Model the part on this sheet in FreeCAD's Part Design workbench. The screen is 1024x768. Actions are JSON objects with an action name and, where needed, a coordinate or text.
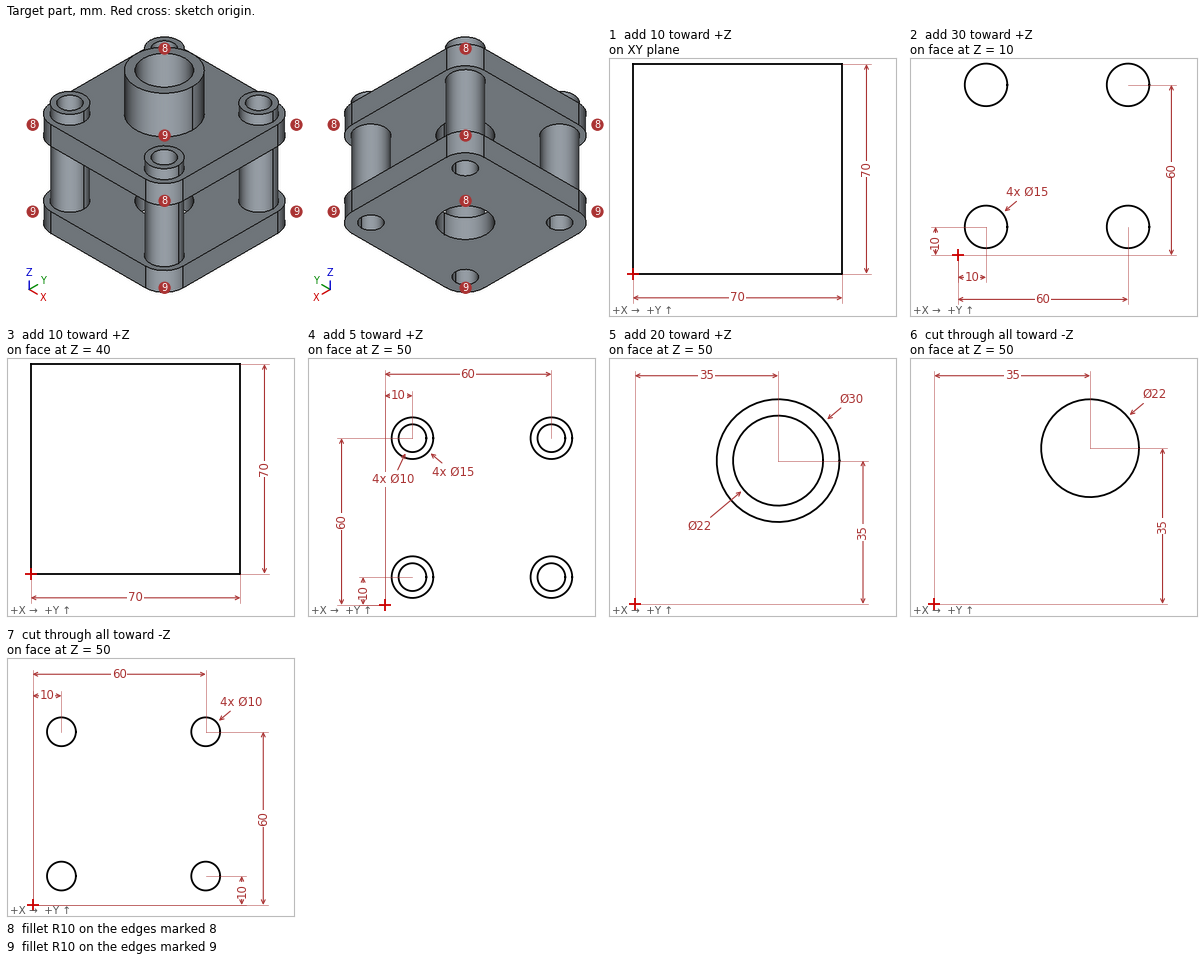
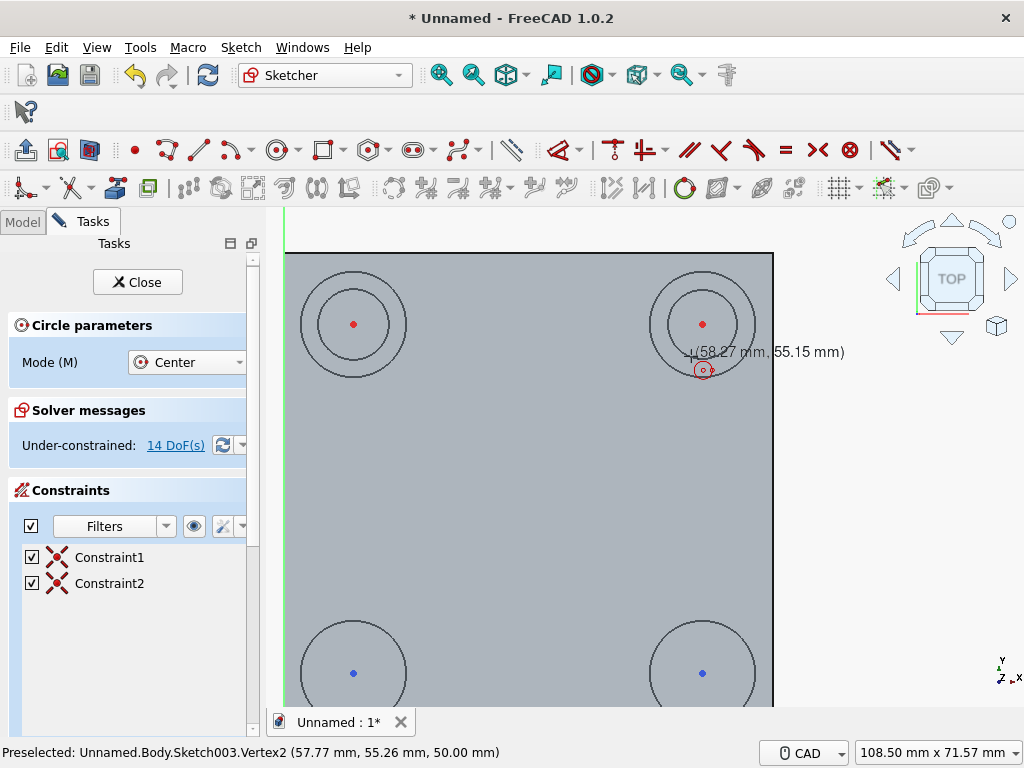
{"action": "left_click", "coordinate": [353, 674]}
{"action": "left_click", "coordinate": [378, 648]}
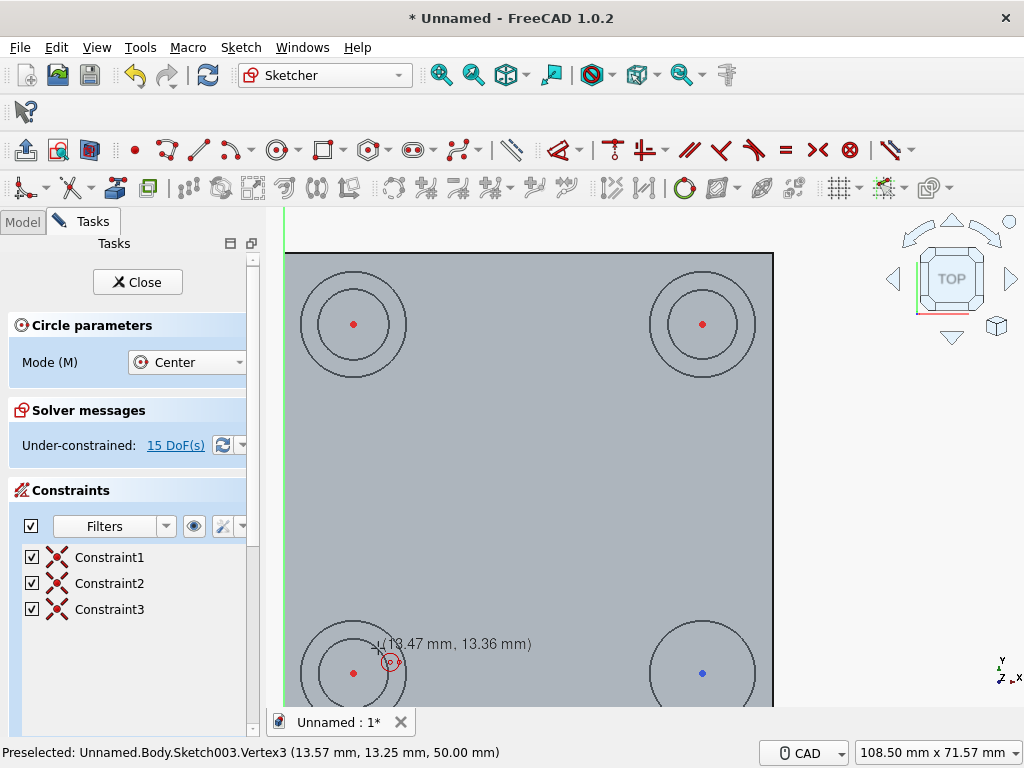
{"action": "left_click", "coordinate": [702, 674]}
{"action": "left_click", "coordinate": [728, 648]}
{"action": "key", "text": "Escape"}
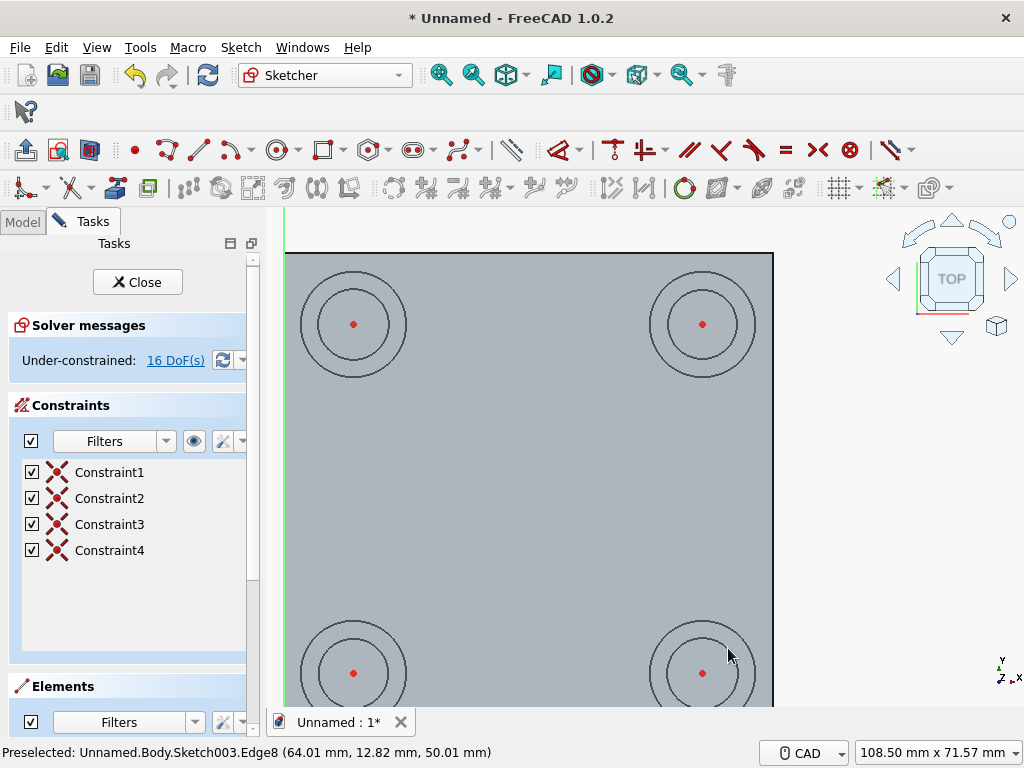
{"action": "left_click", "coordinate": [391, 287]}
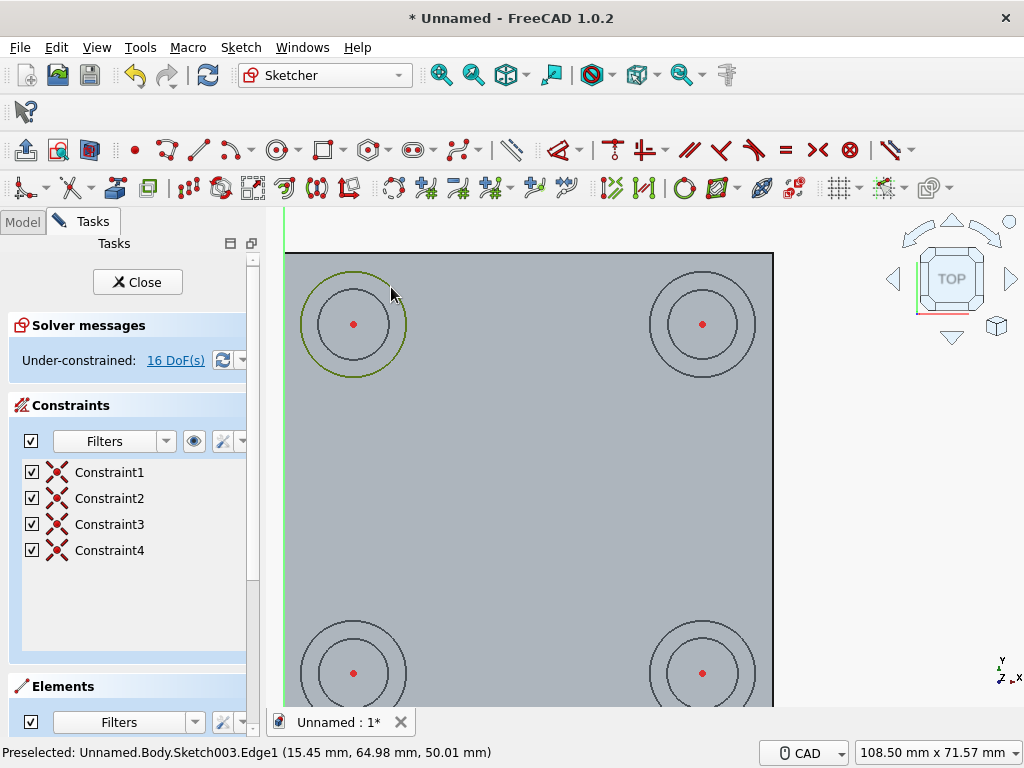
{"action": "left_click", "coordinate": [740, 287]}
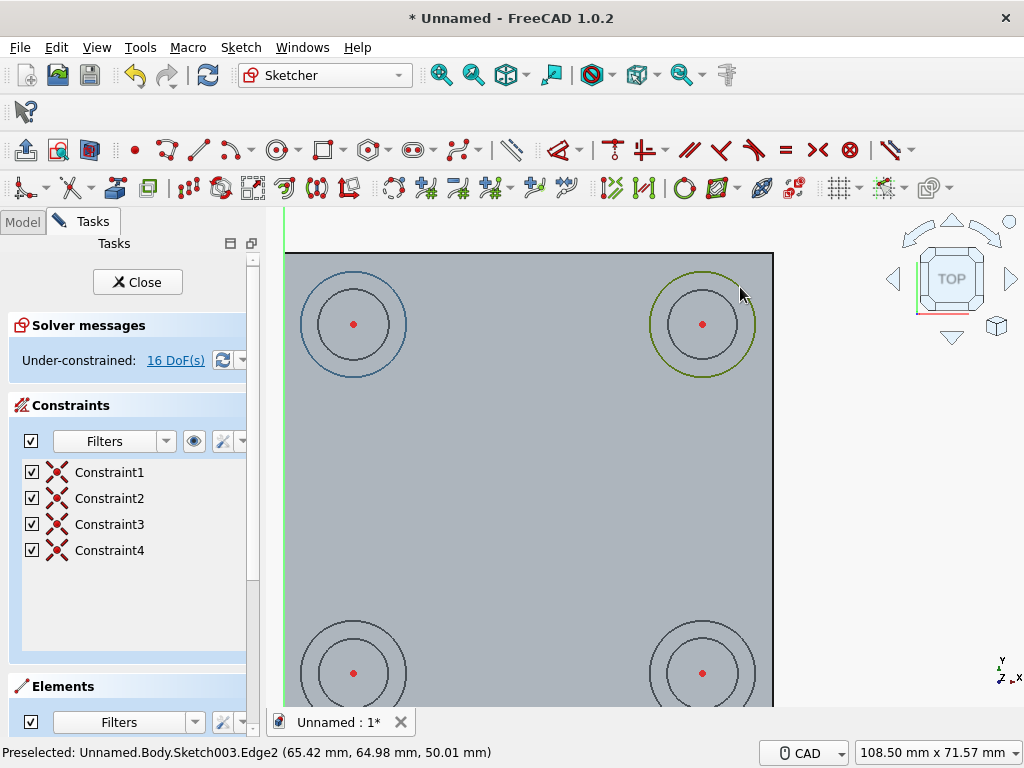
{"action": "left_click", "coordinate": [391, 636]}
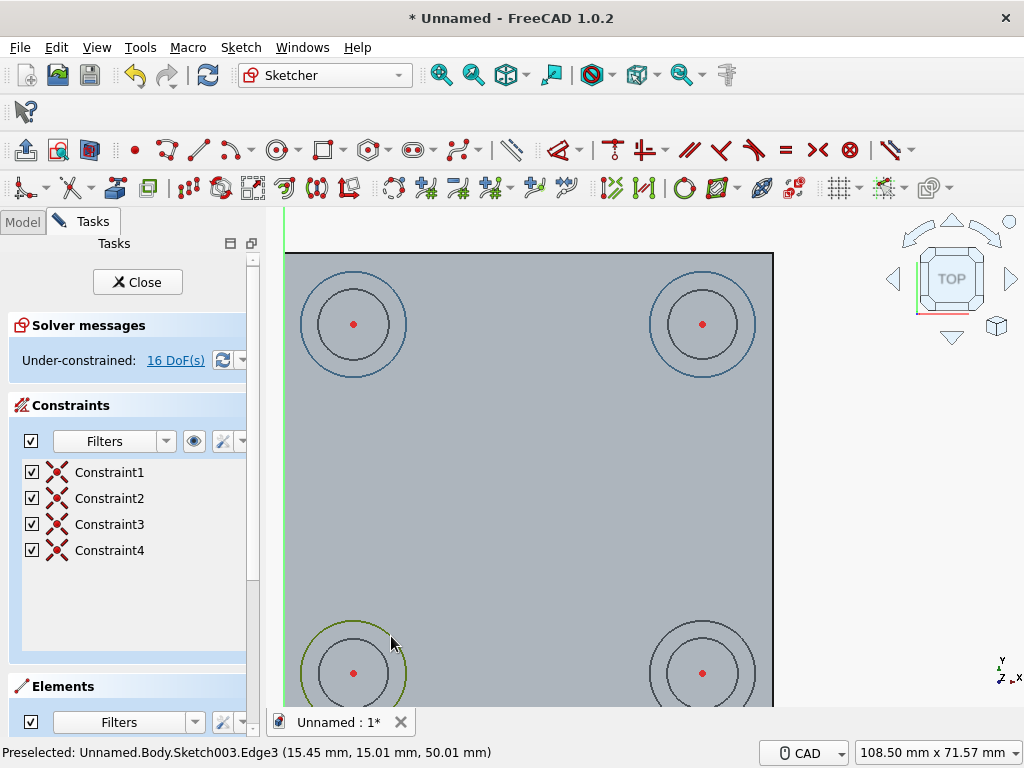
{"action": "left_click", "coordinate": [740, 636]}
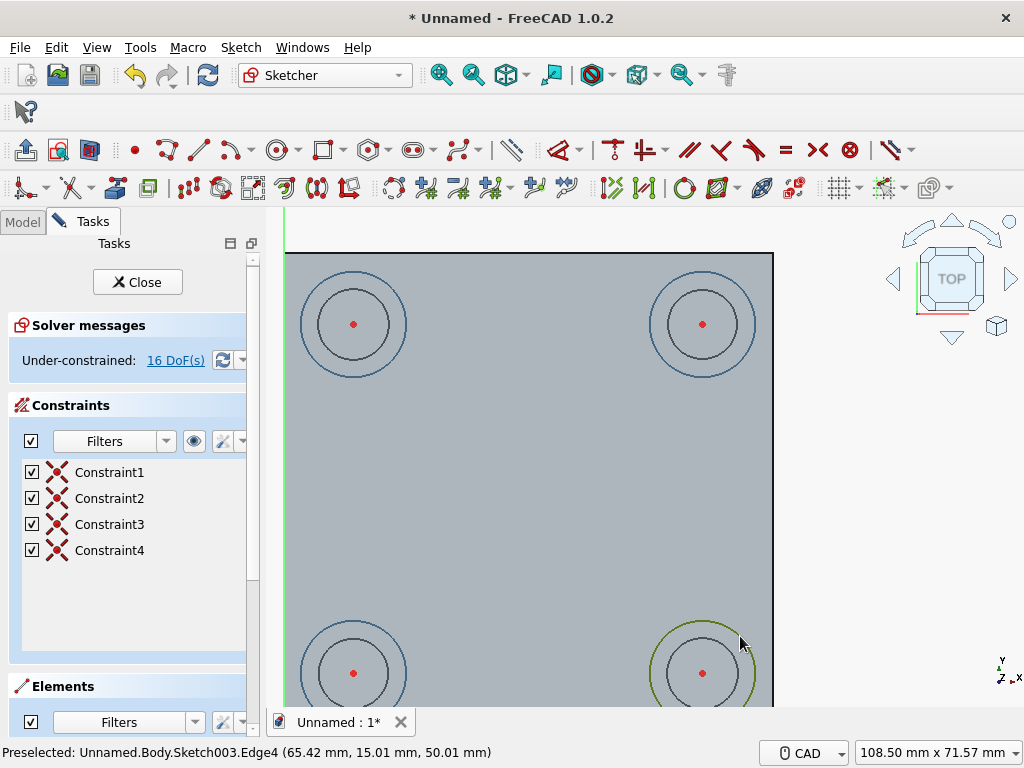
{"action": "left_click", "coordinate": [786, 150]}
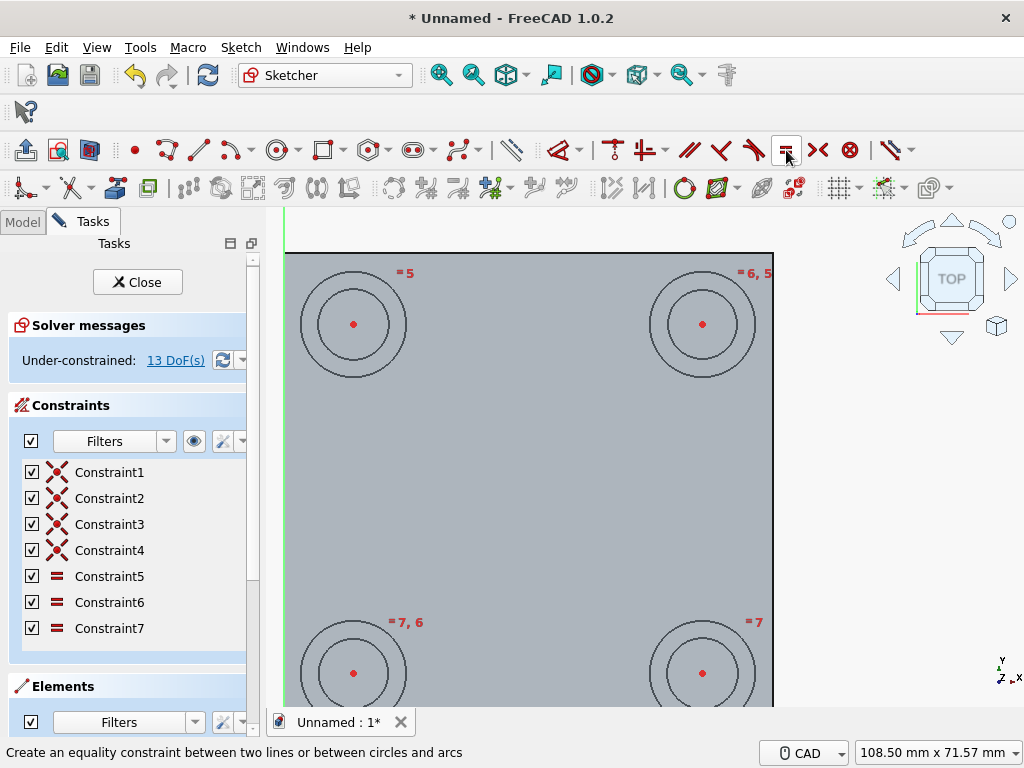
{"action": "left_click", "coordinate": [378, 299]}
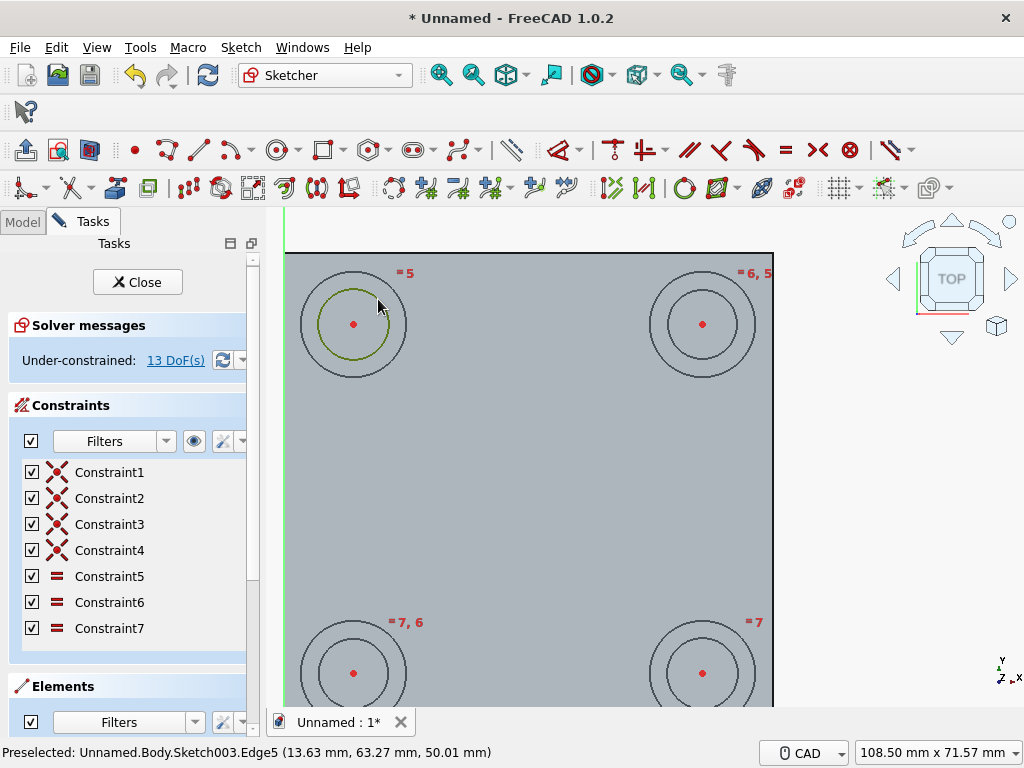
{"action": "left_click", "coordinate": [727, 300]}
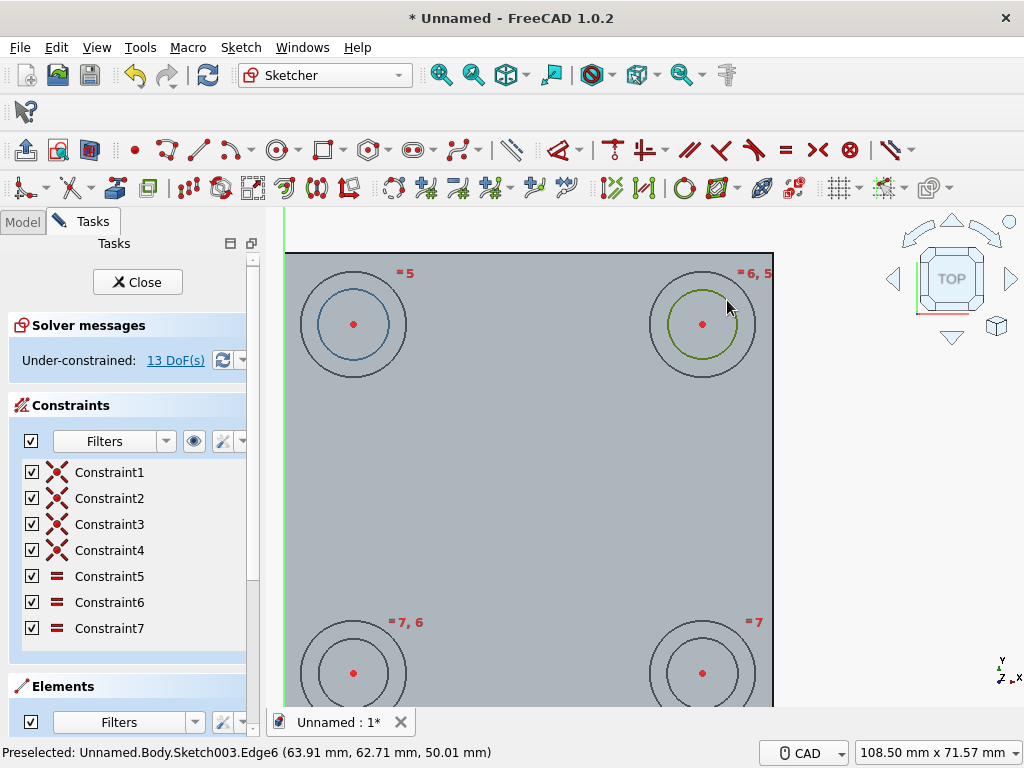
{"action": "left_click", "coordinate": [378, 649]}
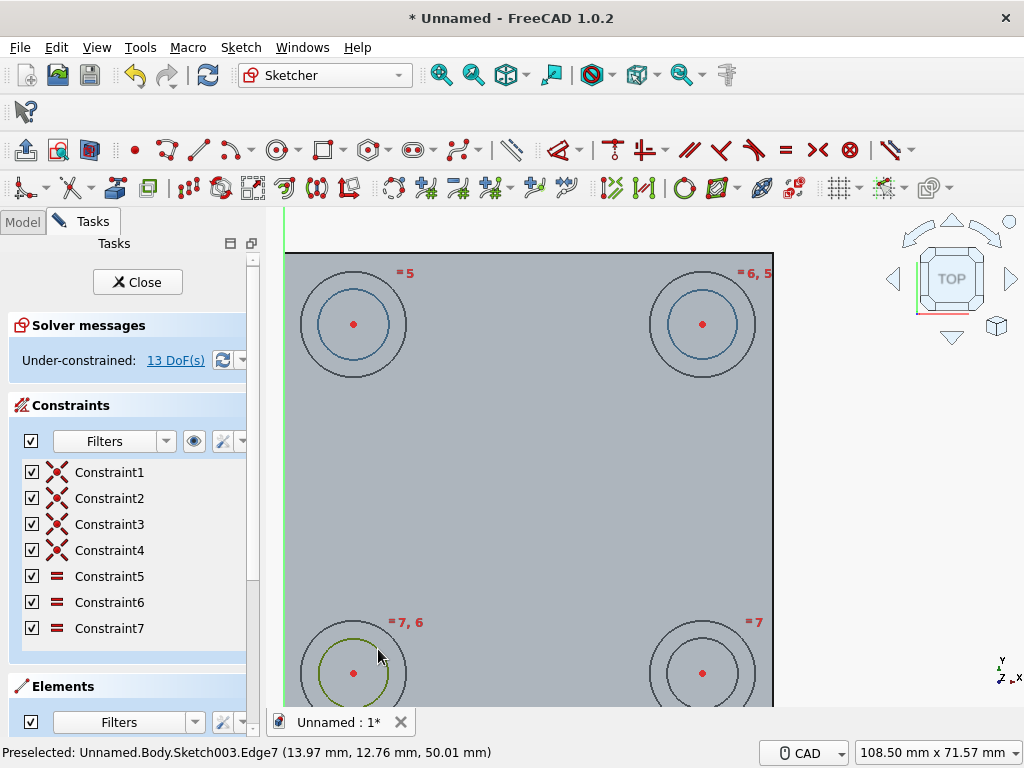
{"action": "left_click", "coordinate": [727, 648]}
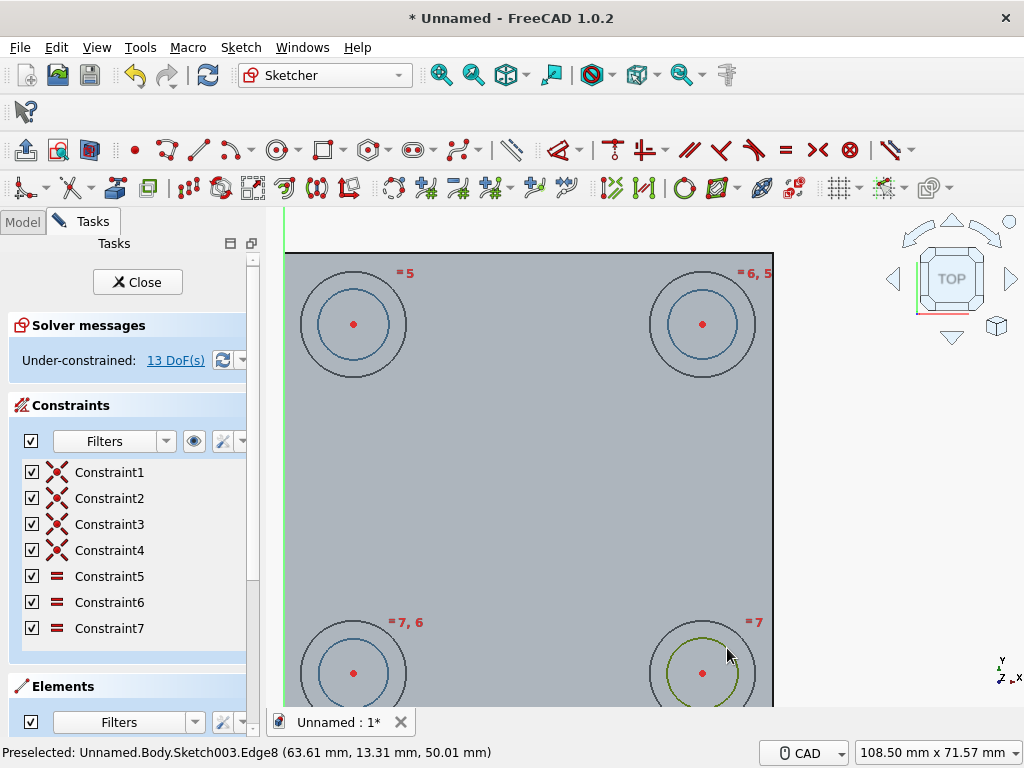
{"action": "key", "text": "e"}